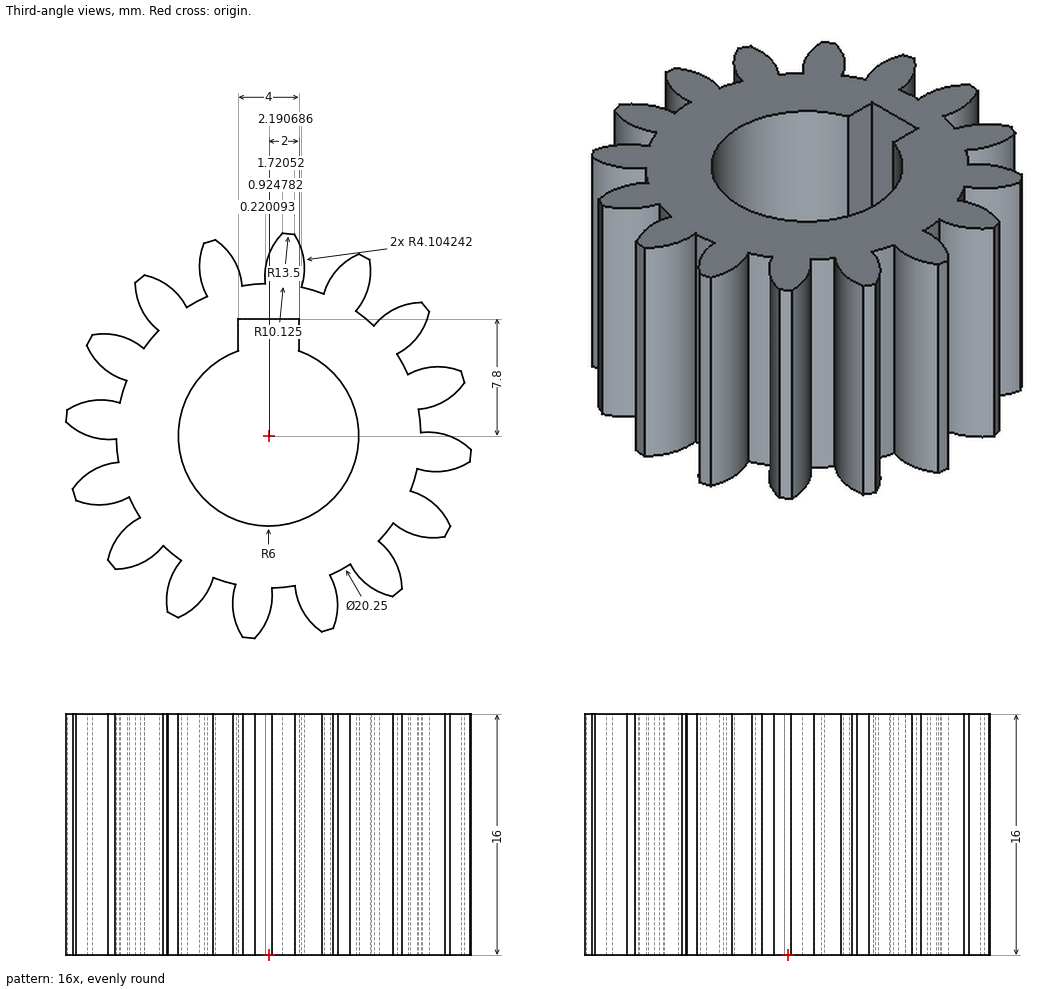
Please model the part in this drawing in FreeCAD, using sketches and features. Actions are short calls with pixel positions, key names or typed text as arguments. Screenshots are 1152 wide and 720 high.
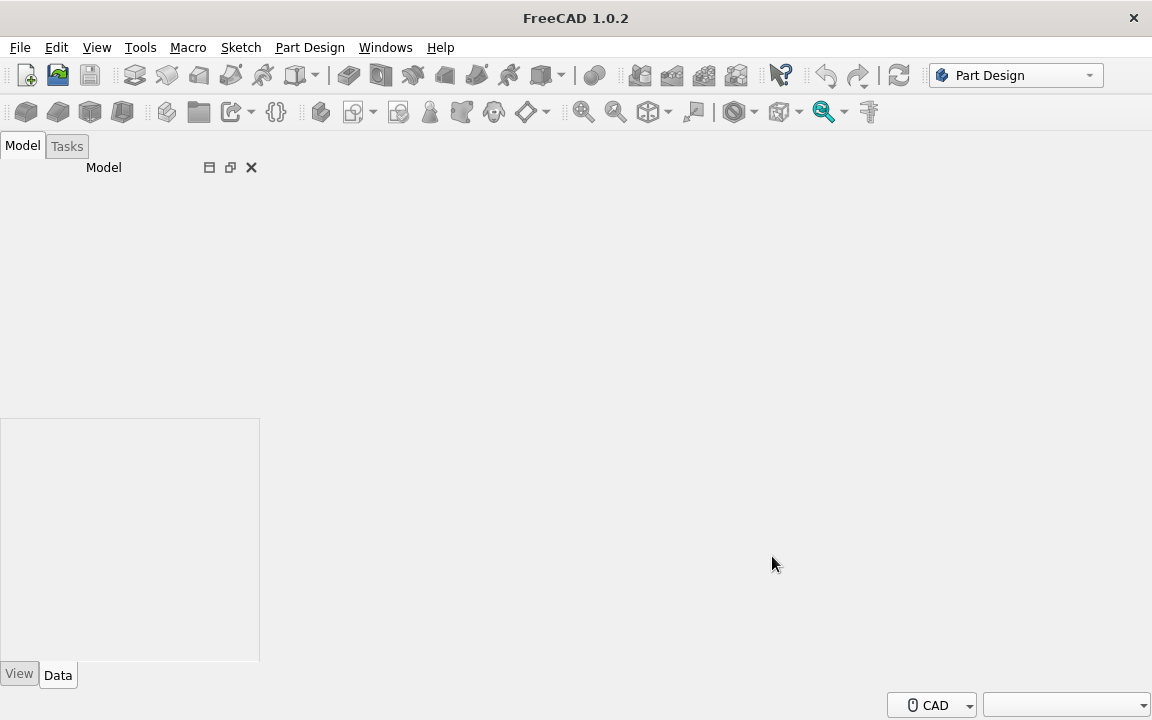
click(26, 76)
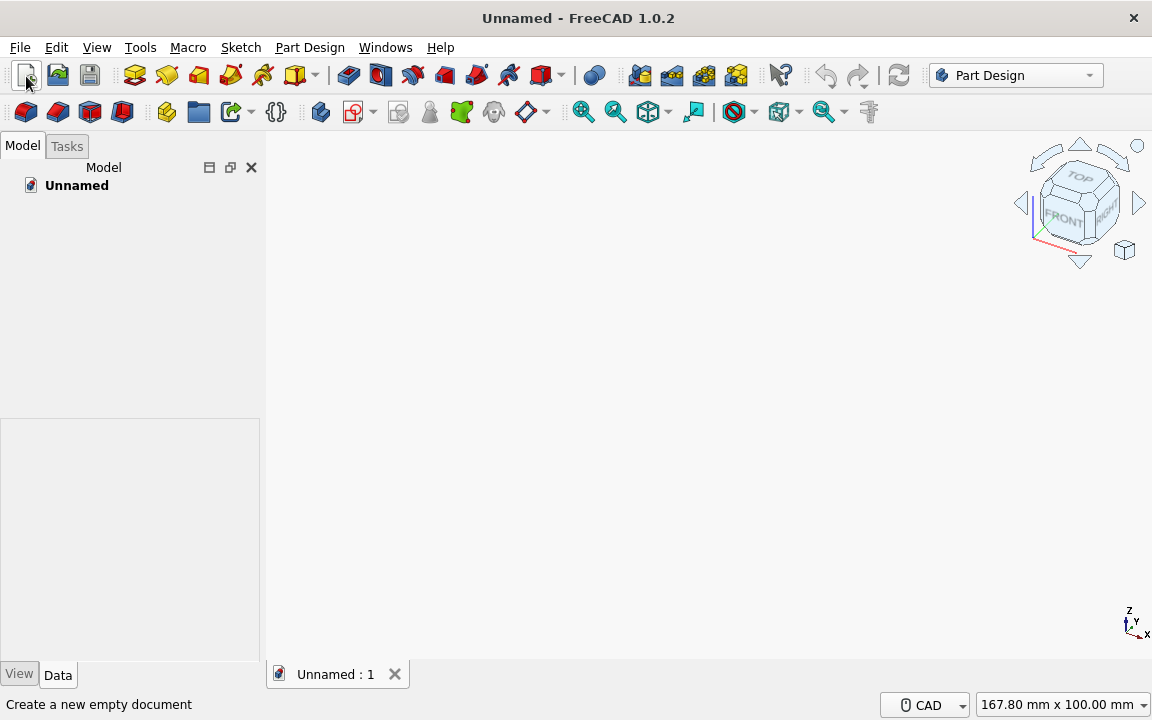
click(354, 112)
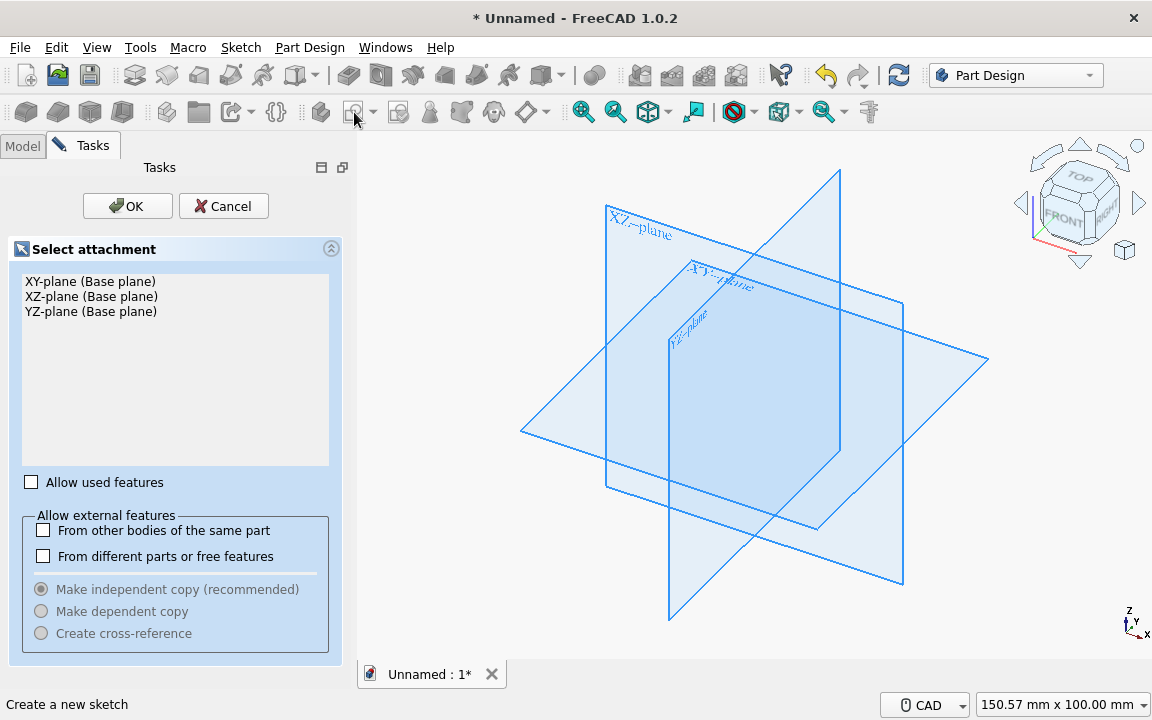
click(82, 282)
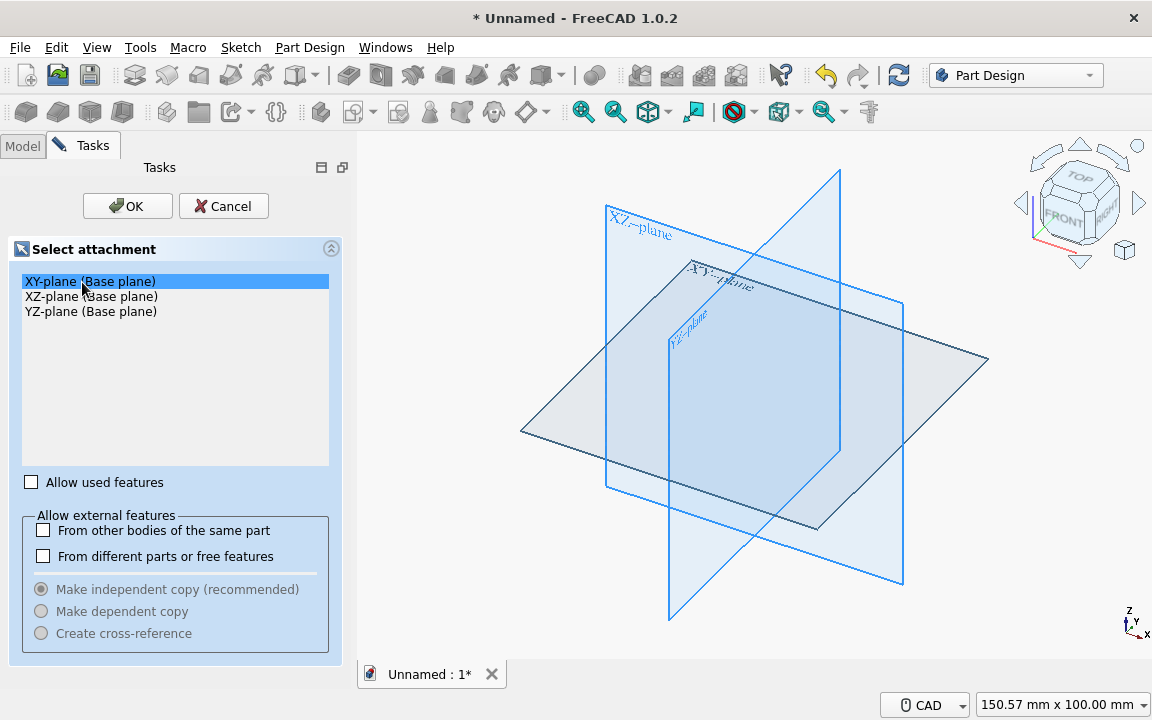
click(128, 206)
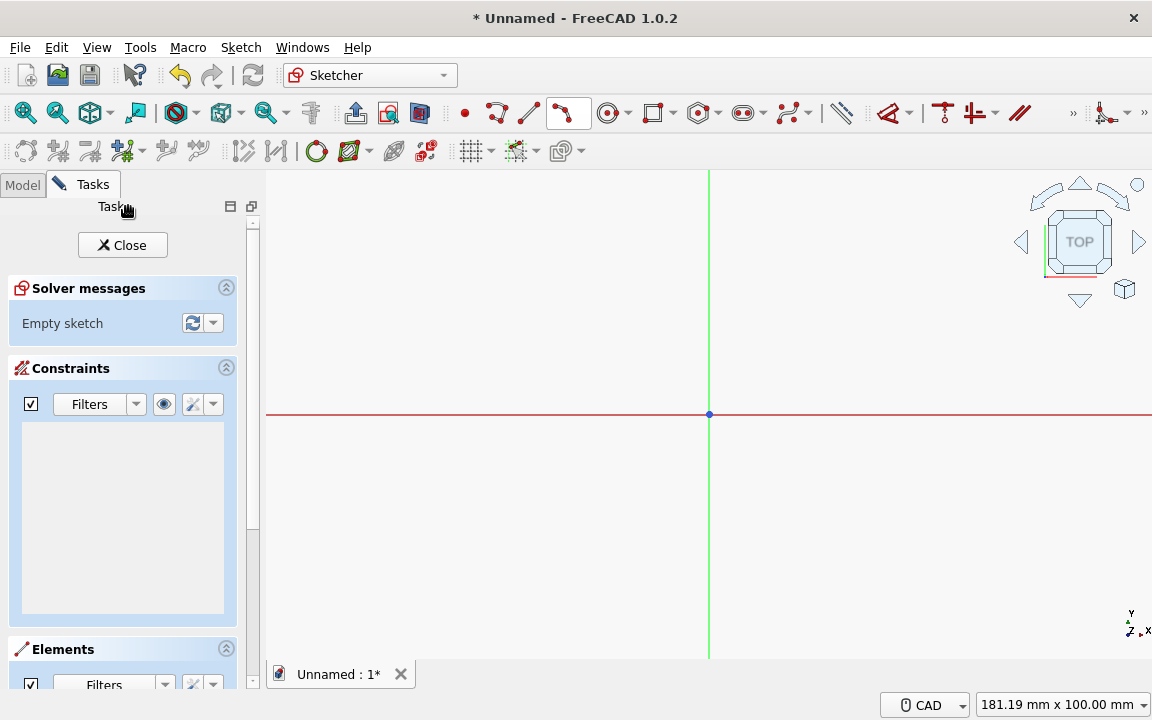
scroll(739, 415, up, 6)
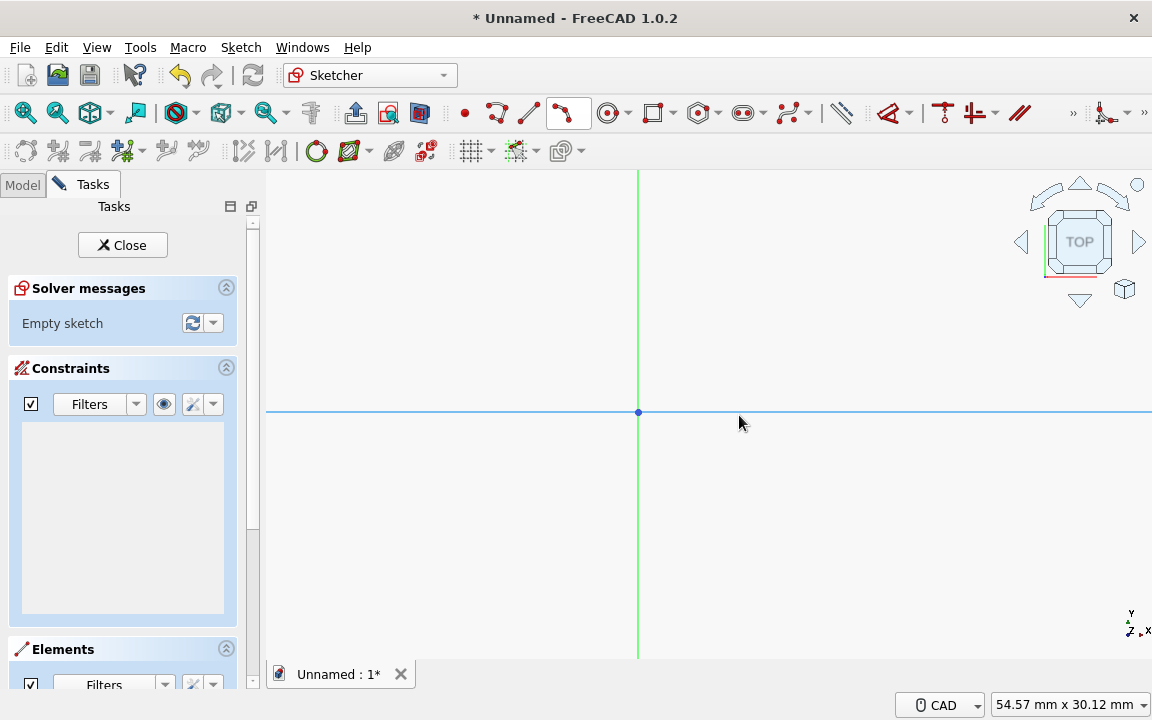
click(608, 114)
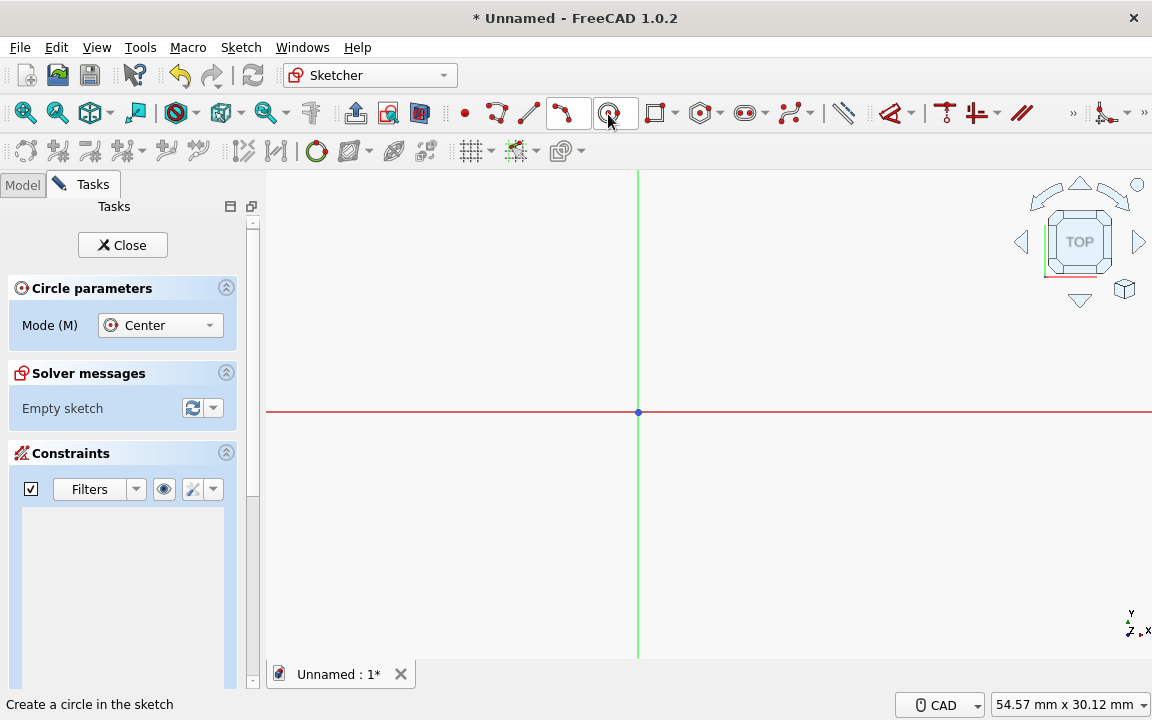
click(638, 412)
move(754, 296)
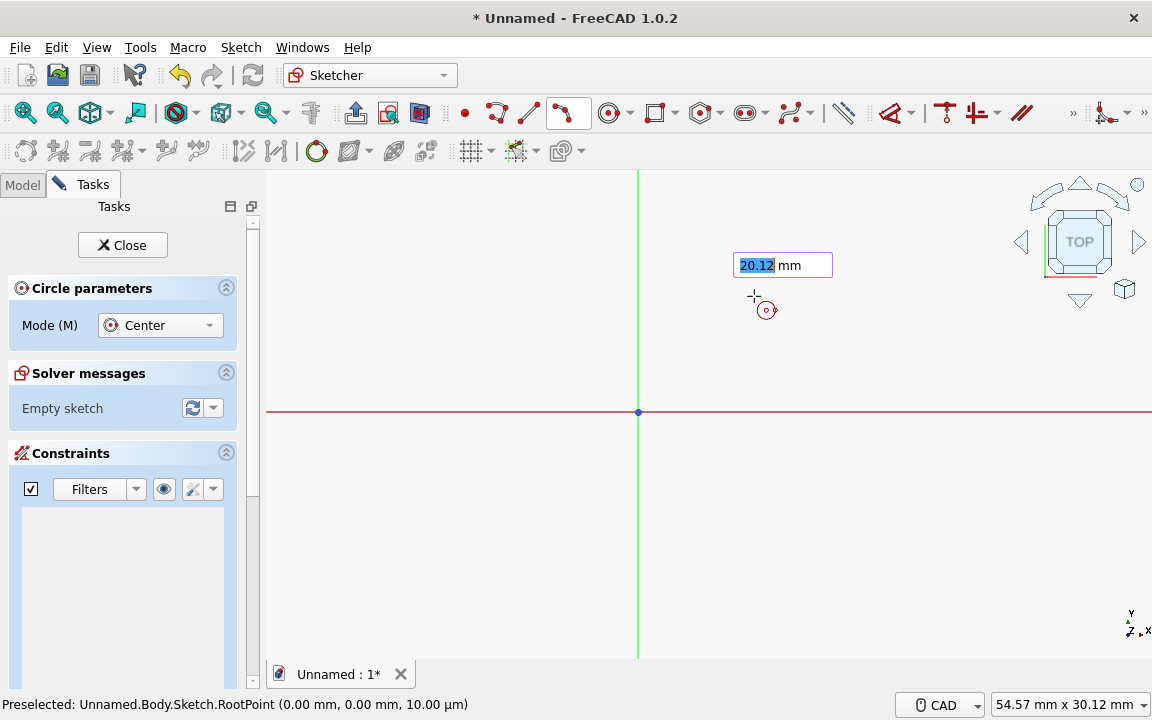
text(20.25)
key(Return)
key(Escape)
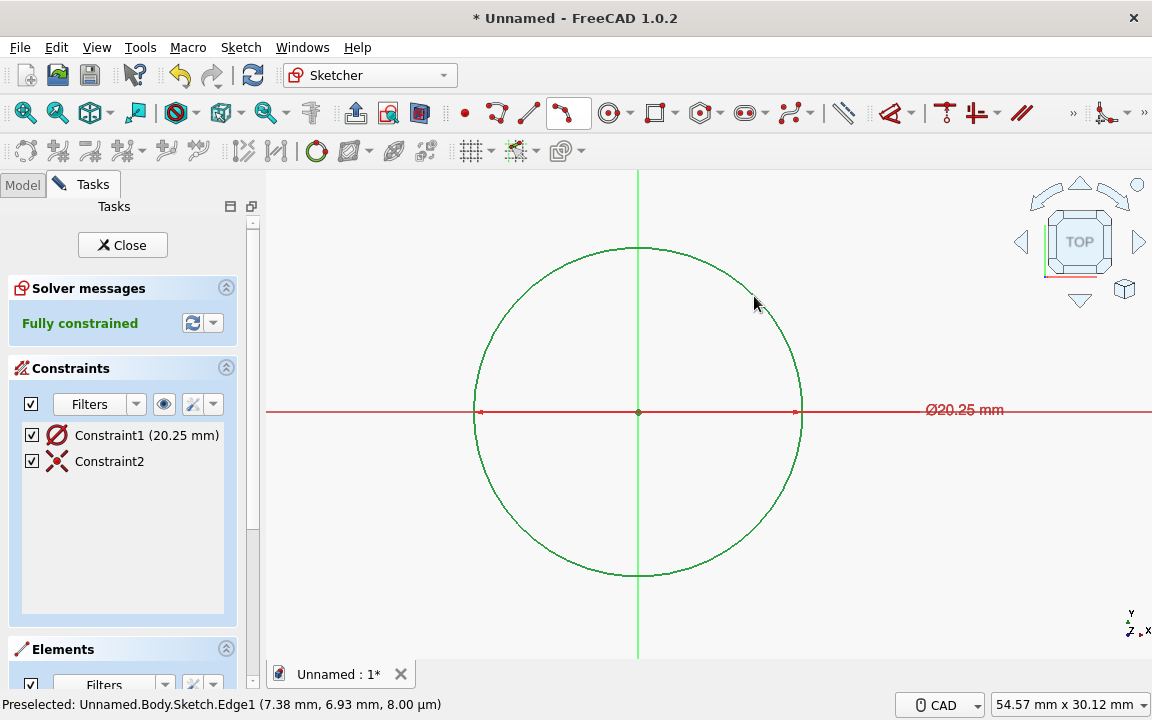
click(123, 245)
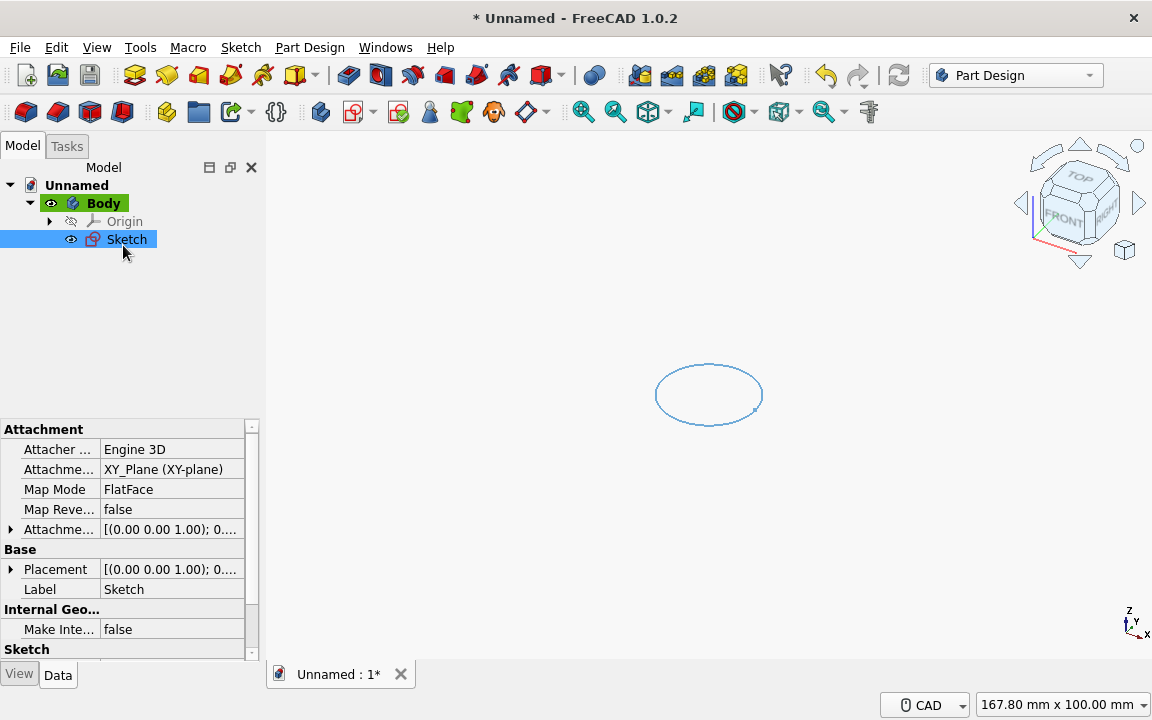
click(136, 76)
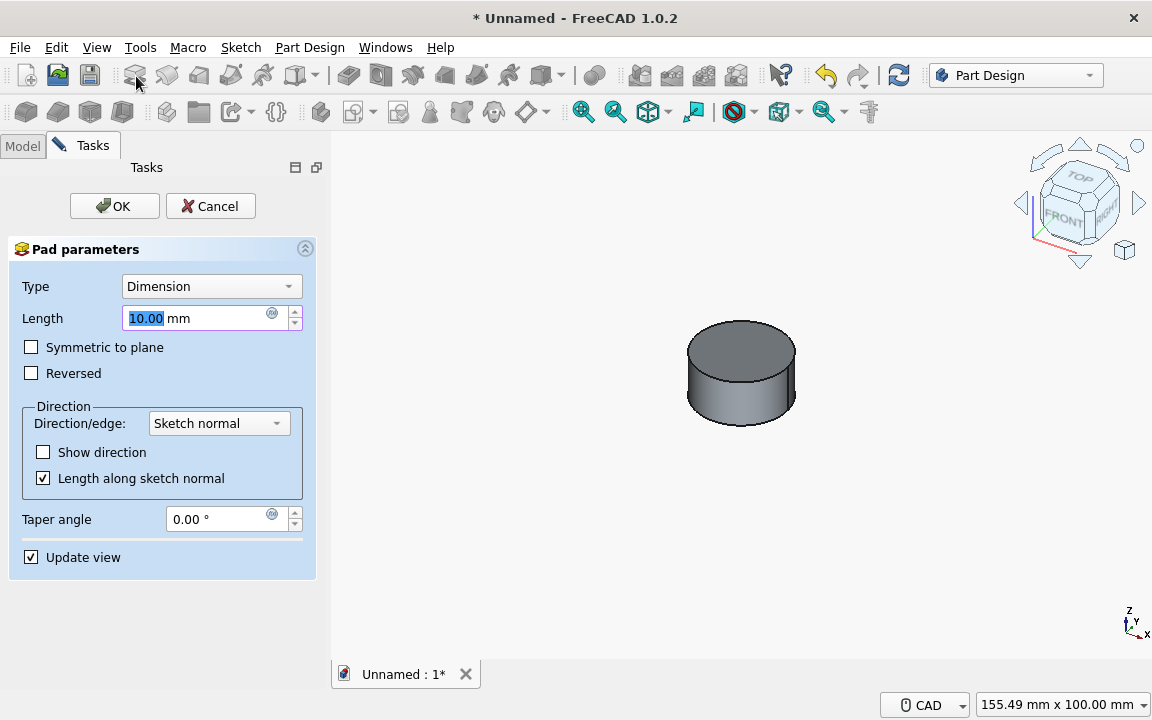
text(16)
key(Tab)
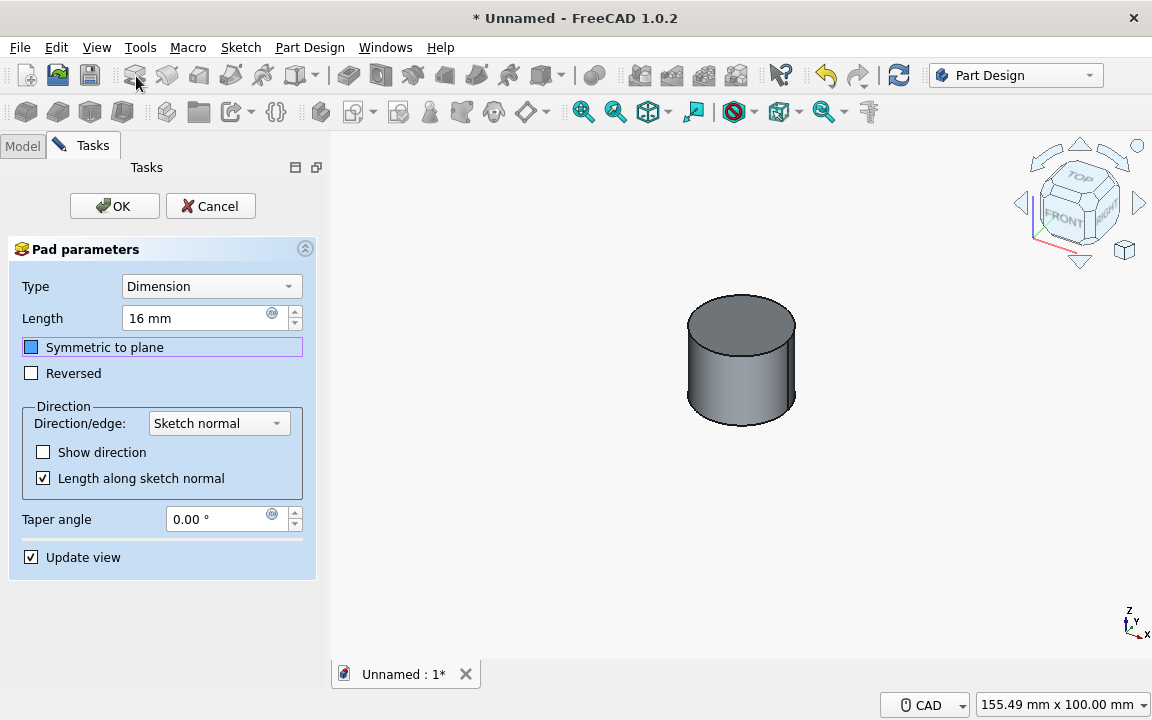
click(115, 206)